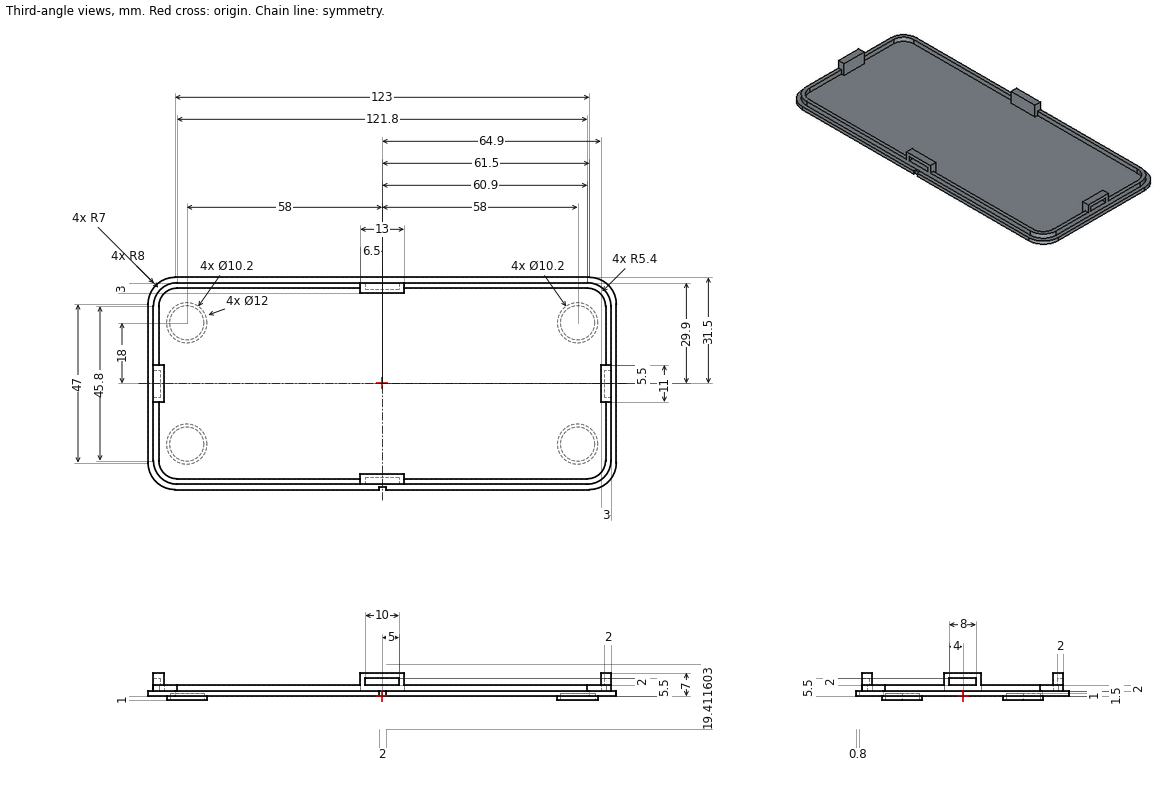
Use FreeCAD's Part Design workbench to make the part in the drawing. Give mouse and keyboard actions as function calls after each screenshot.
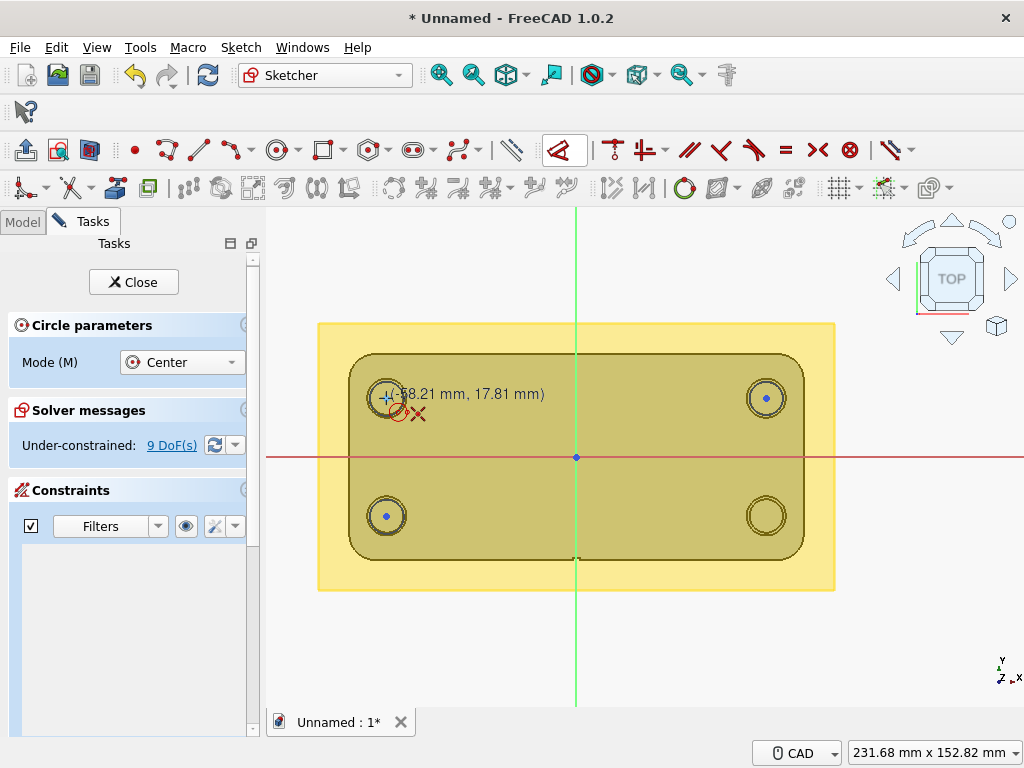
scroll(766, 516, up, 2)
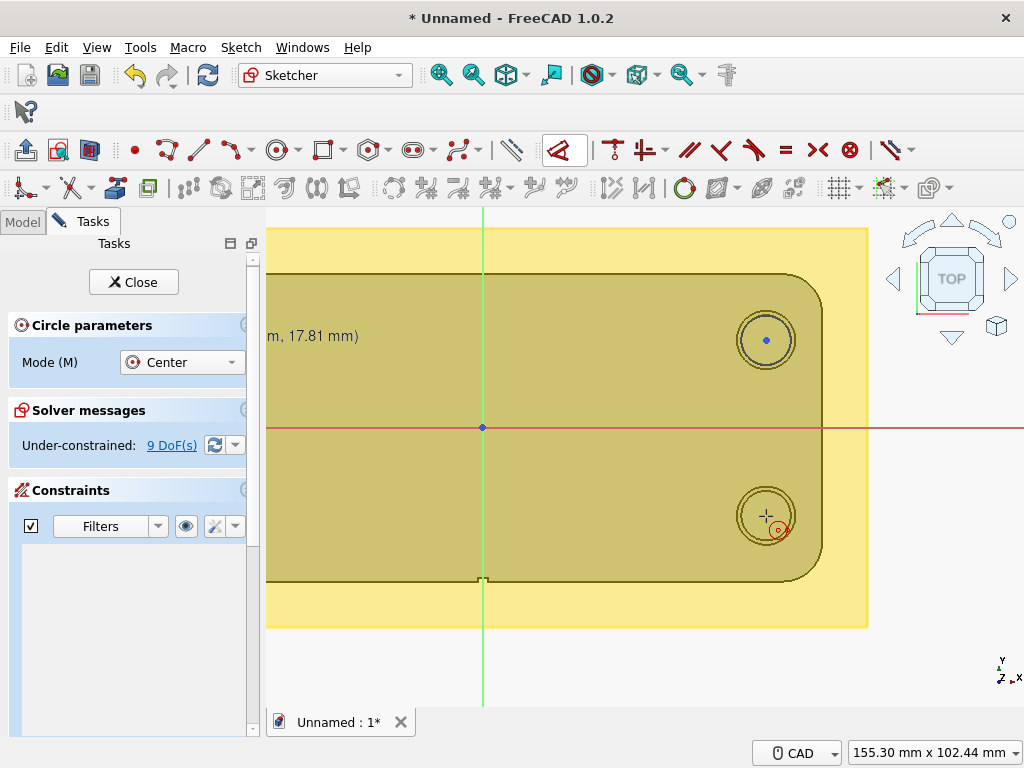
click(766, 516)
click(784, 498)
key(Escape)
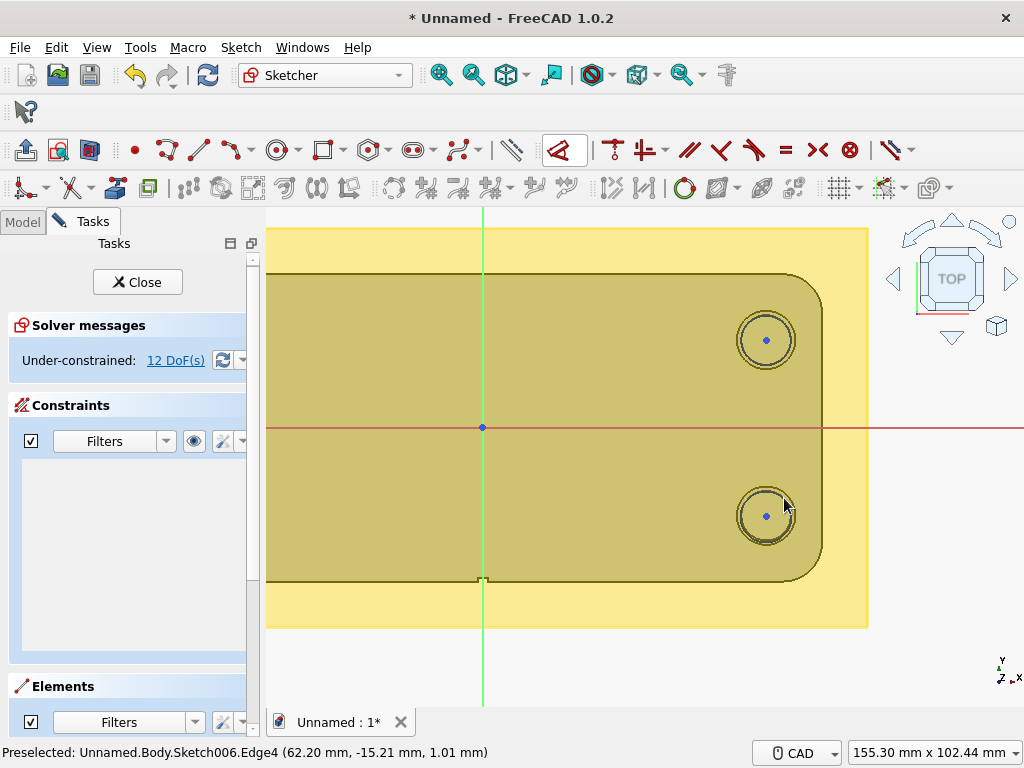
click(783, 323)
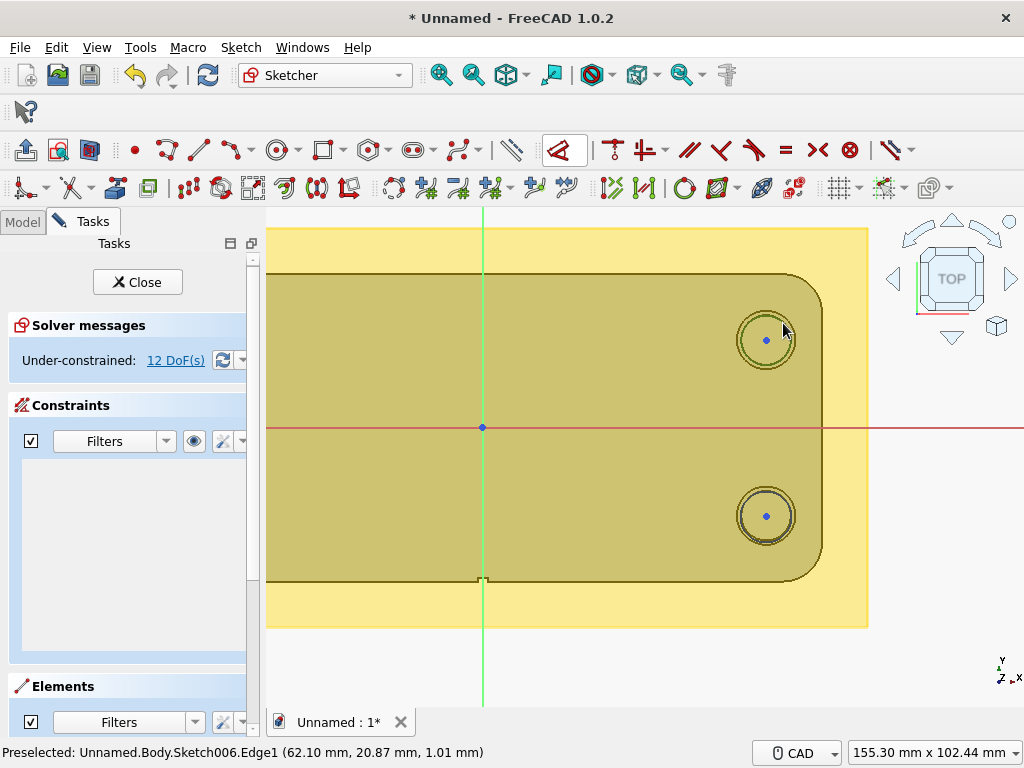
scroll(767, 516, down, 2)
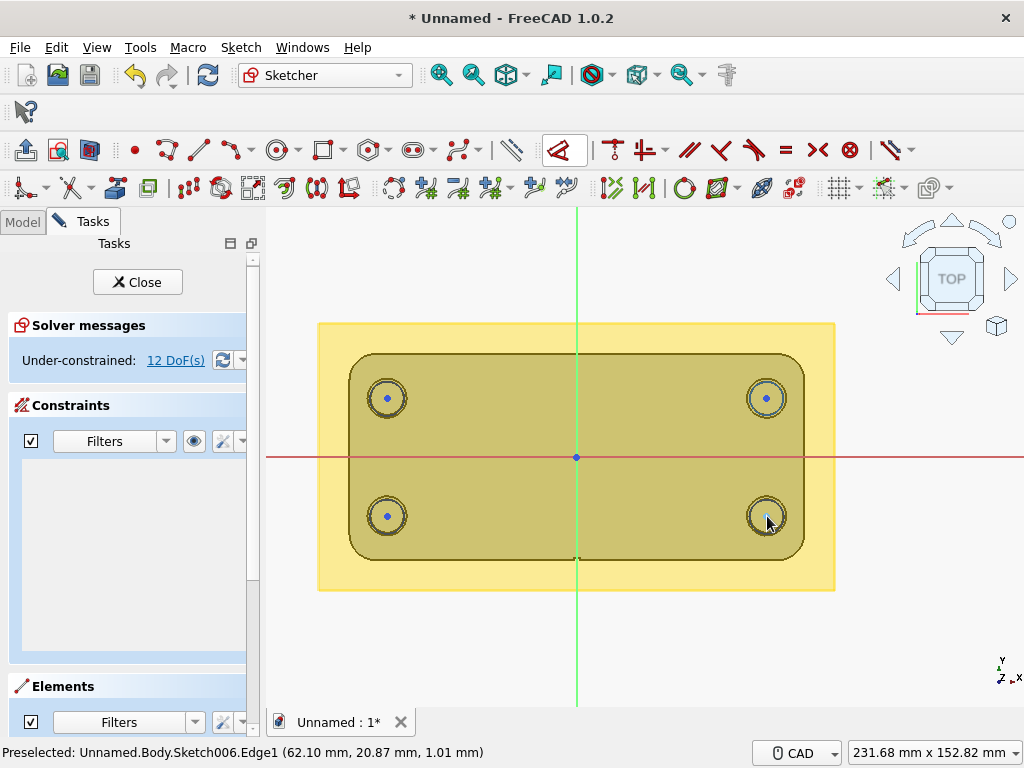
click(399, 387)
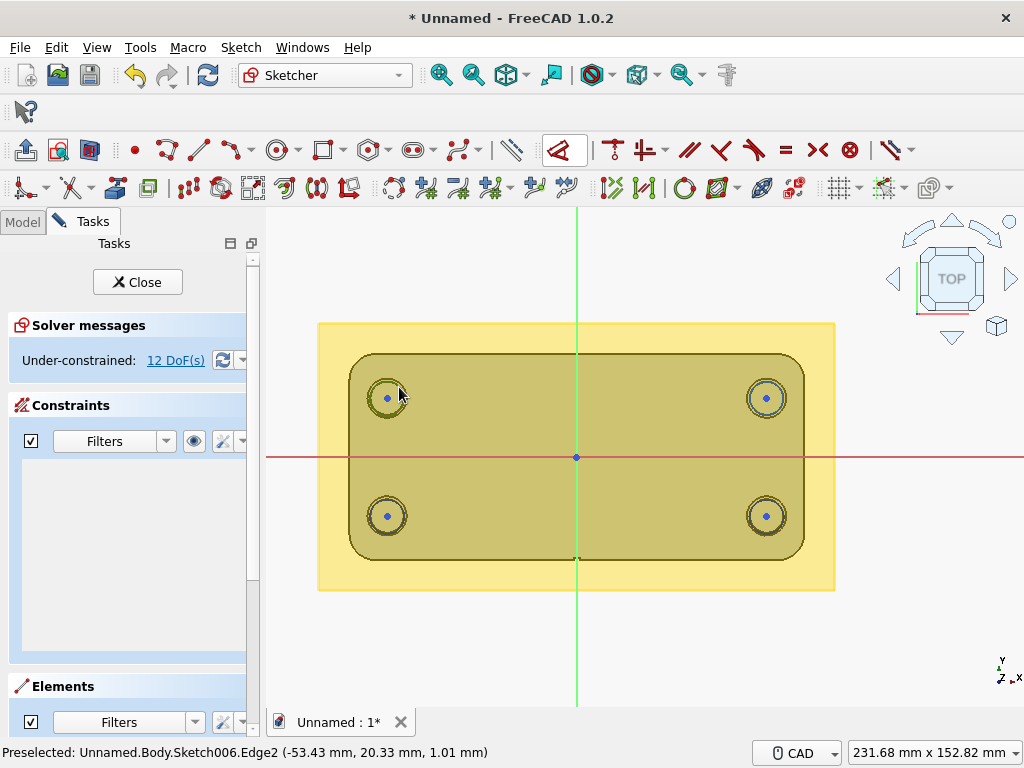
click(399, 505)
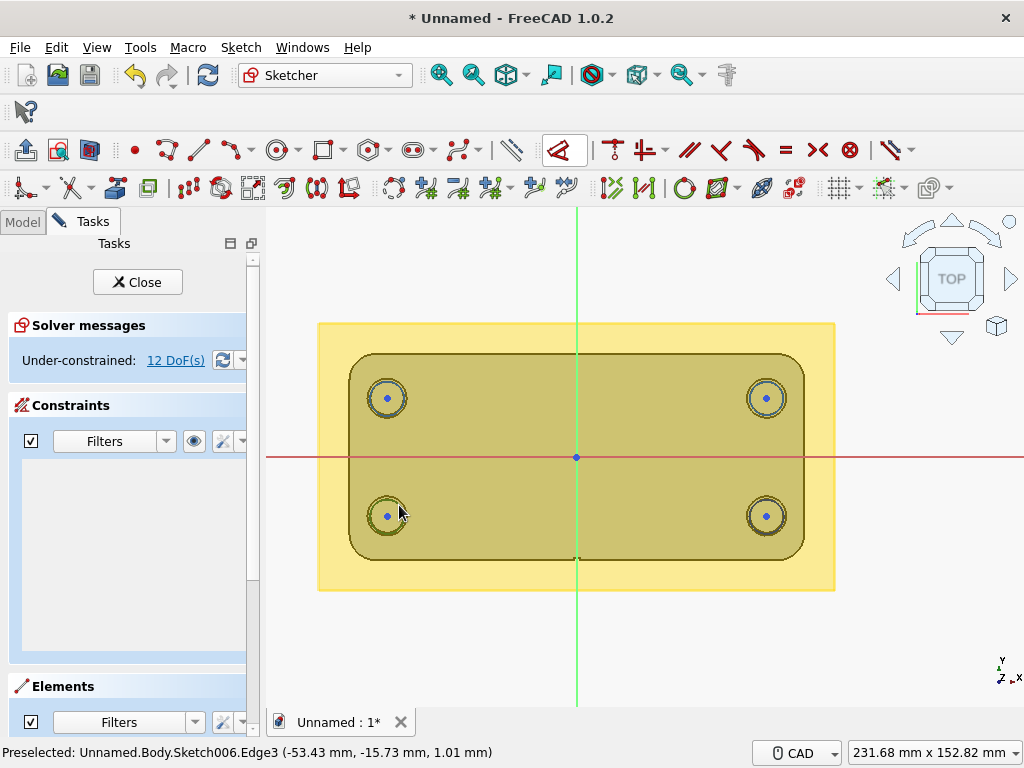
click(779, 505)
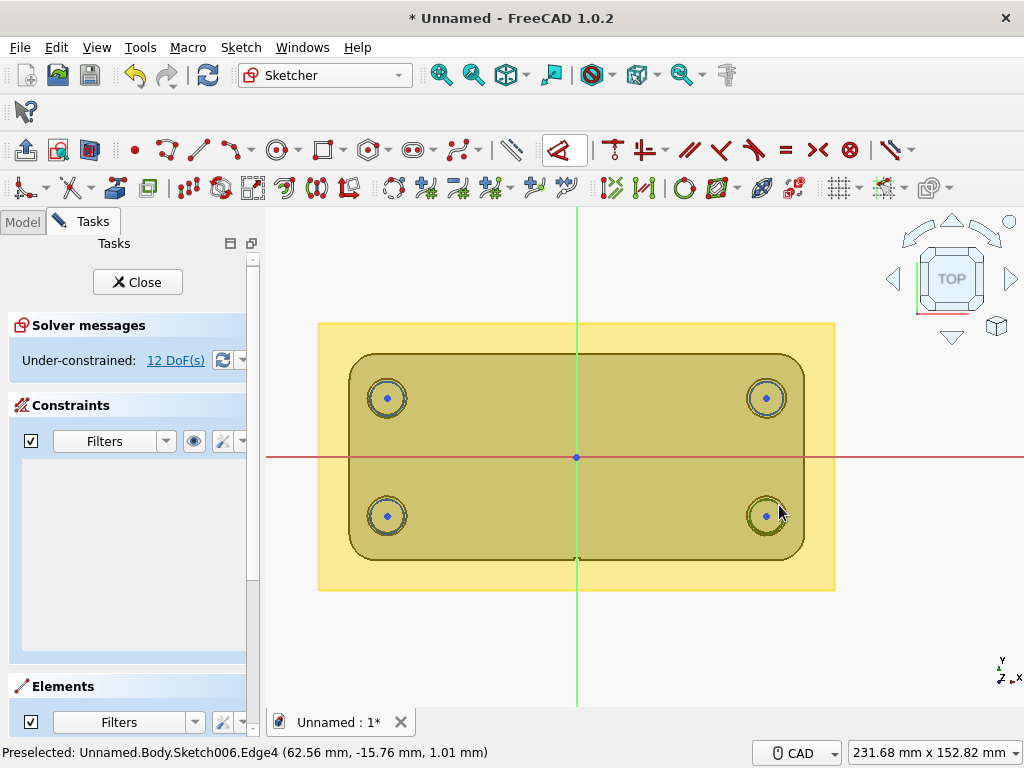
key(e)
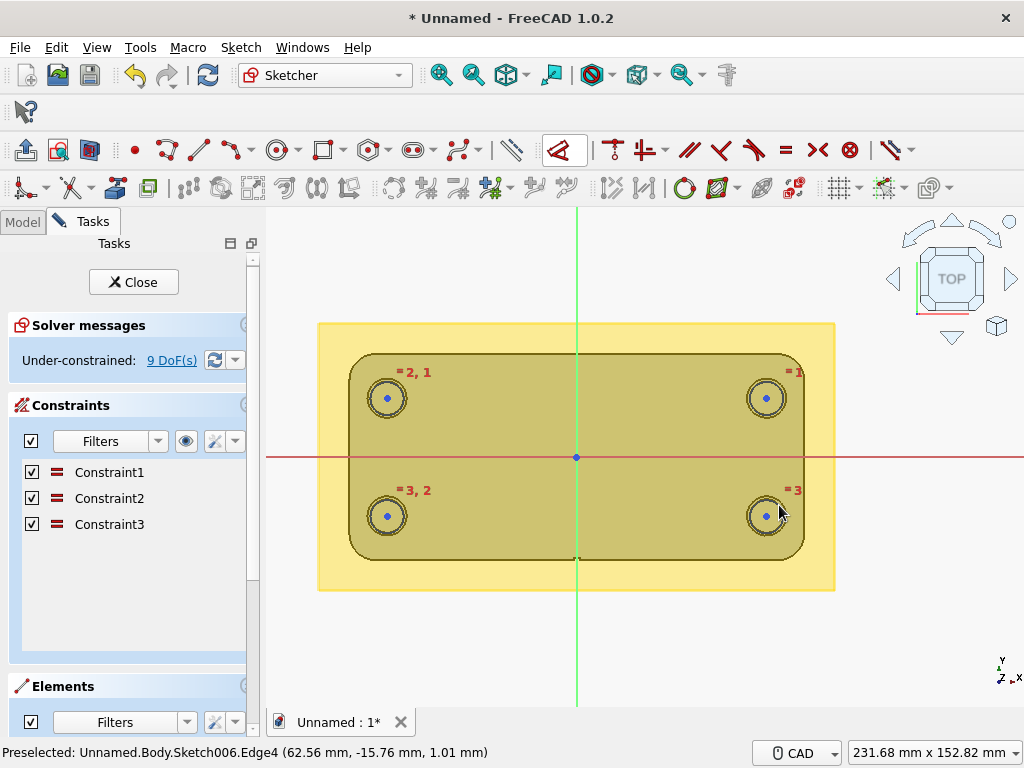
click(767, 399)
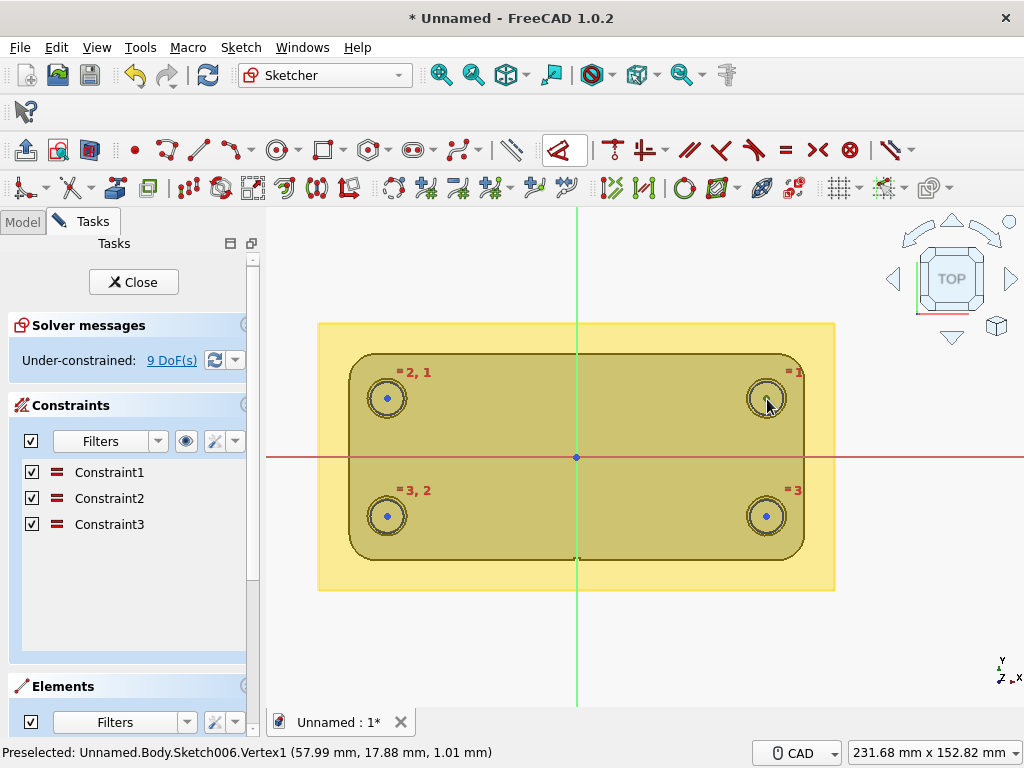
click(387, 399)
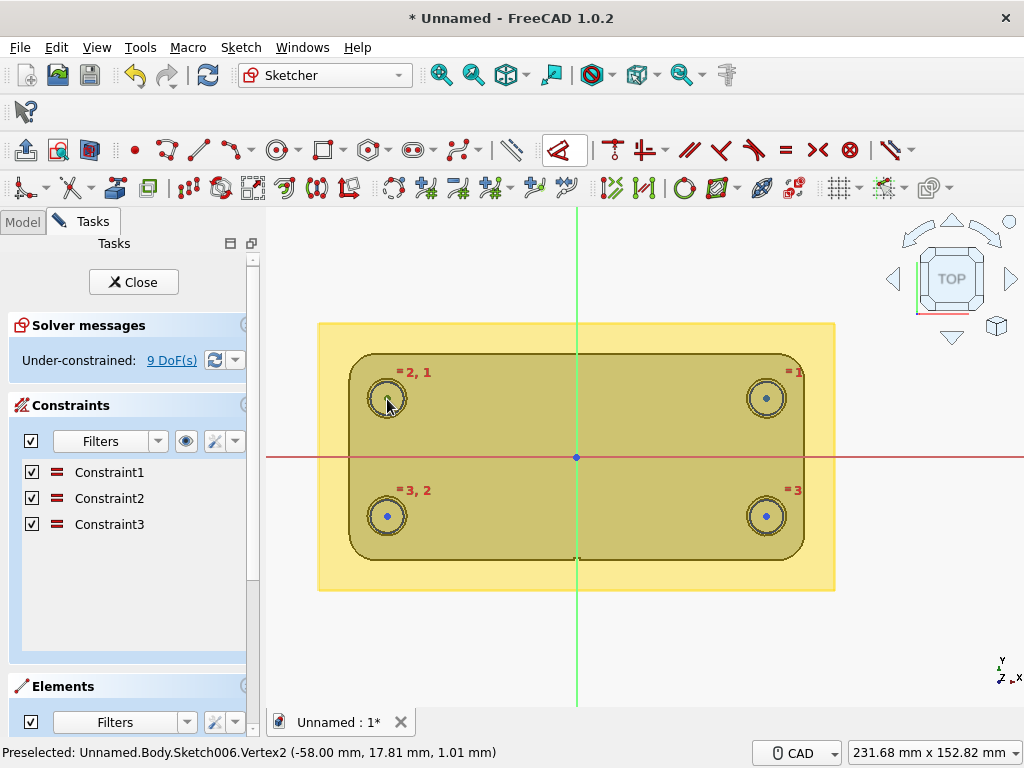
click(577, 647)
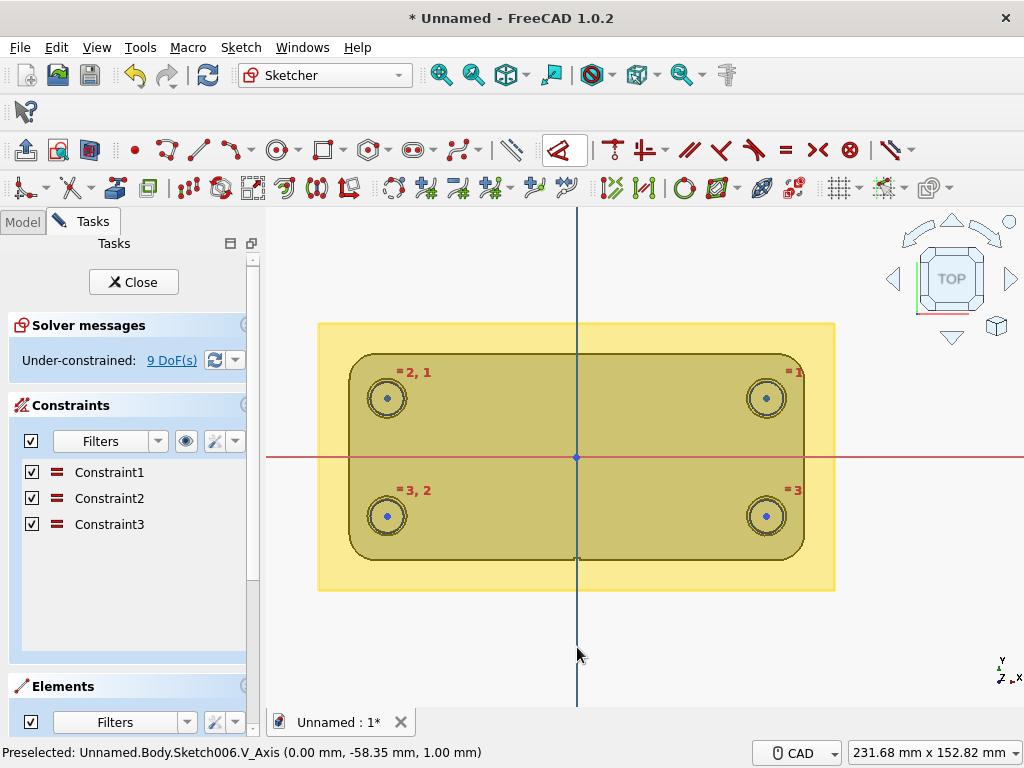
click(818, 150)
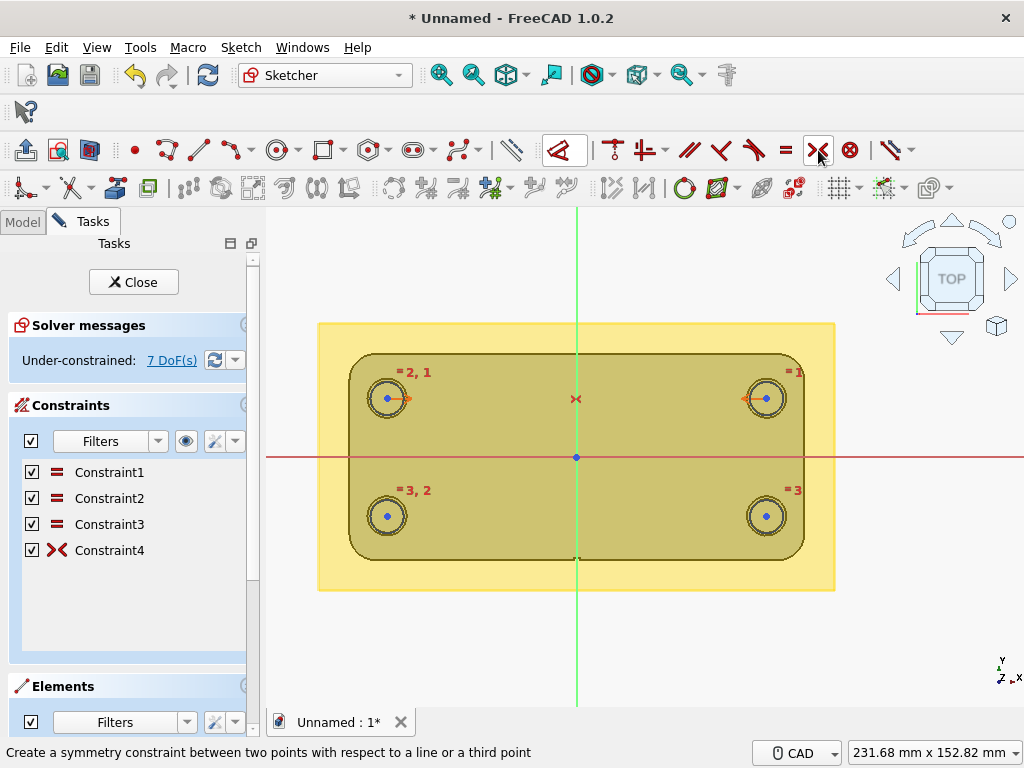
click(387, 399)